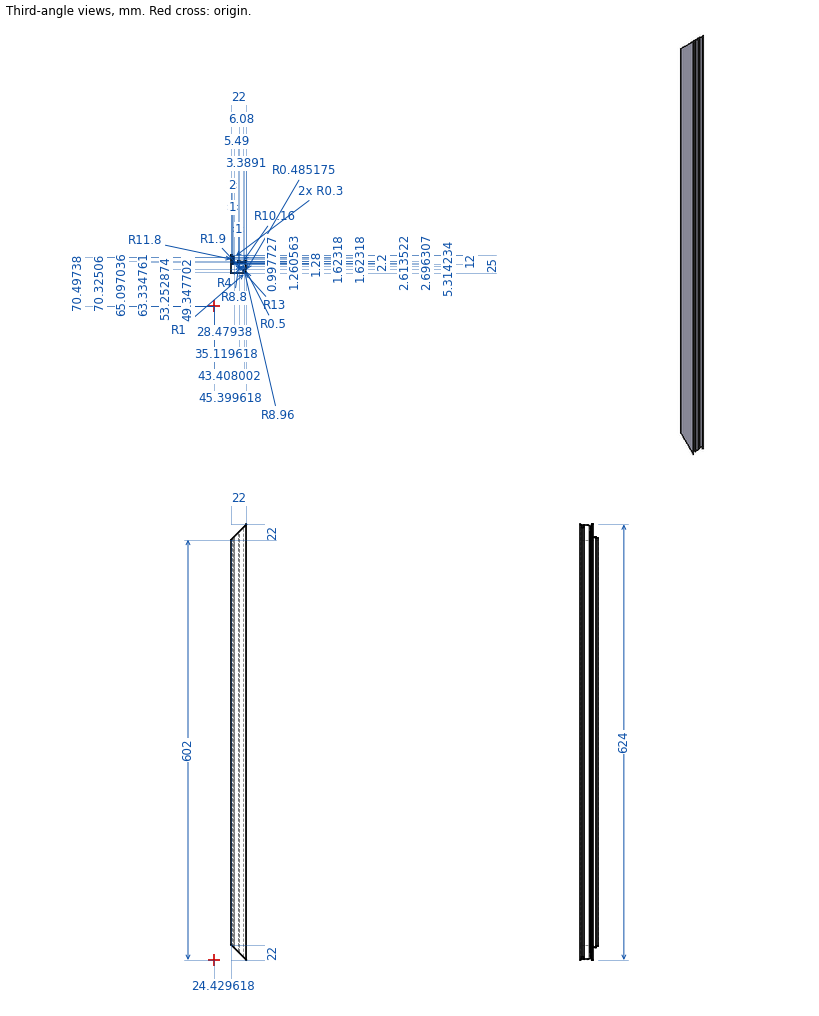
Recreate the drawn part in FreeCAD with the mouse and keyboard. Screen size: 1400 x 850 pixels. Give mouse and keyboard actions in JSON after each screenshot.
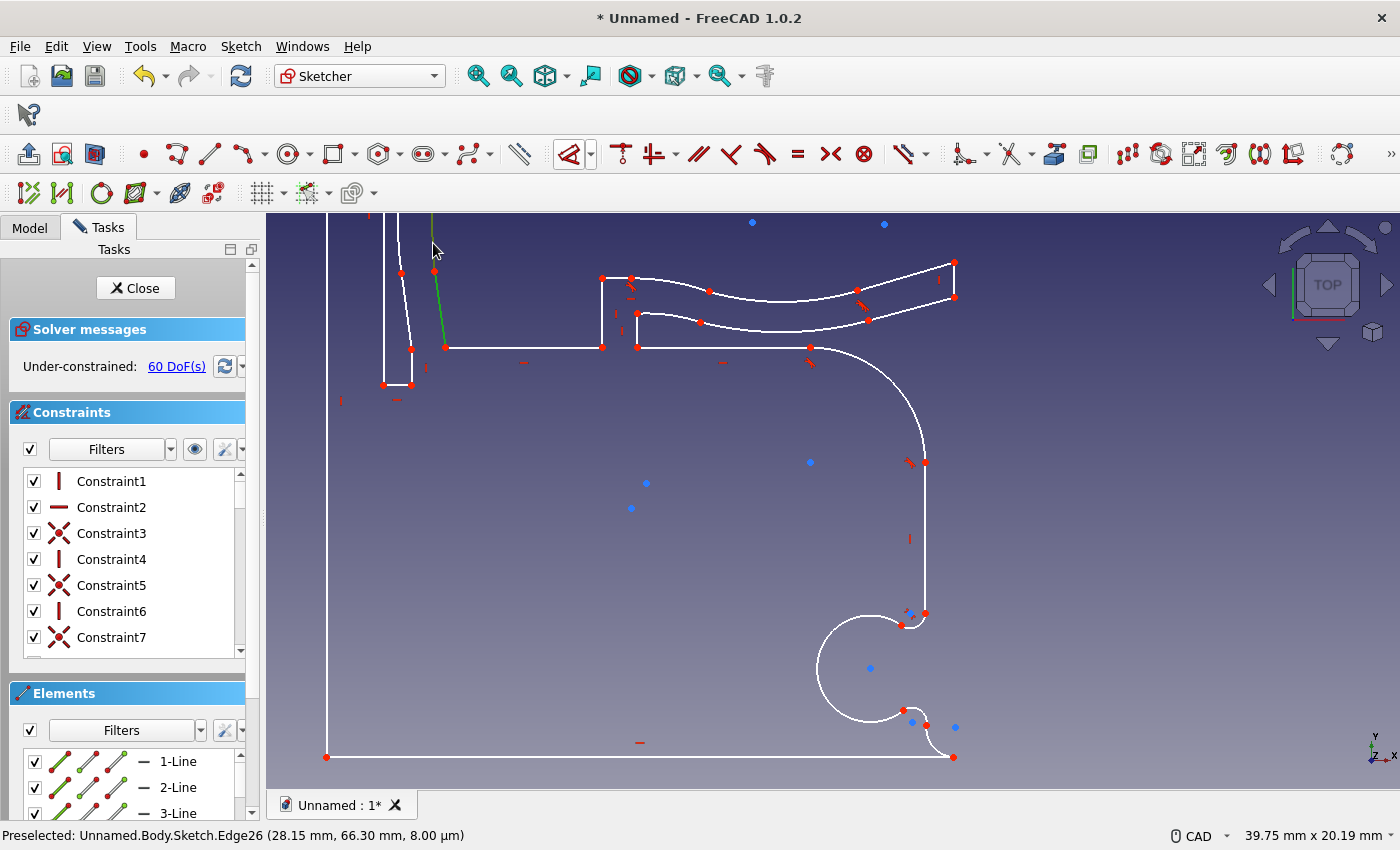
{"action": "left_click", "coordinate": [765, 154]}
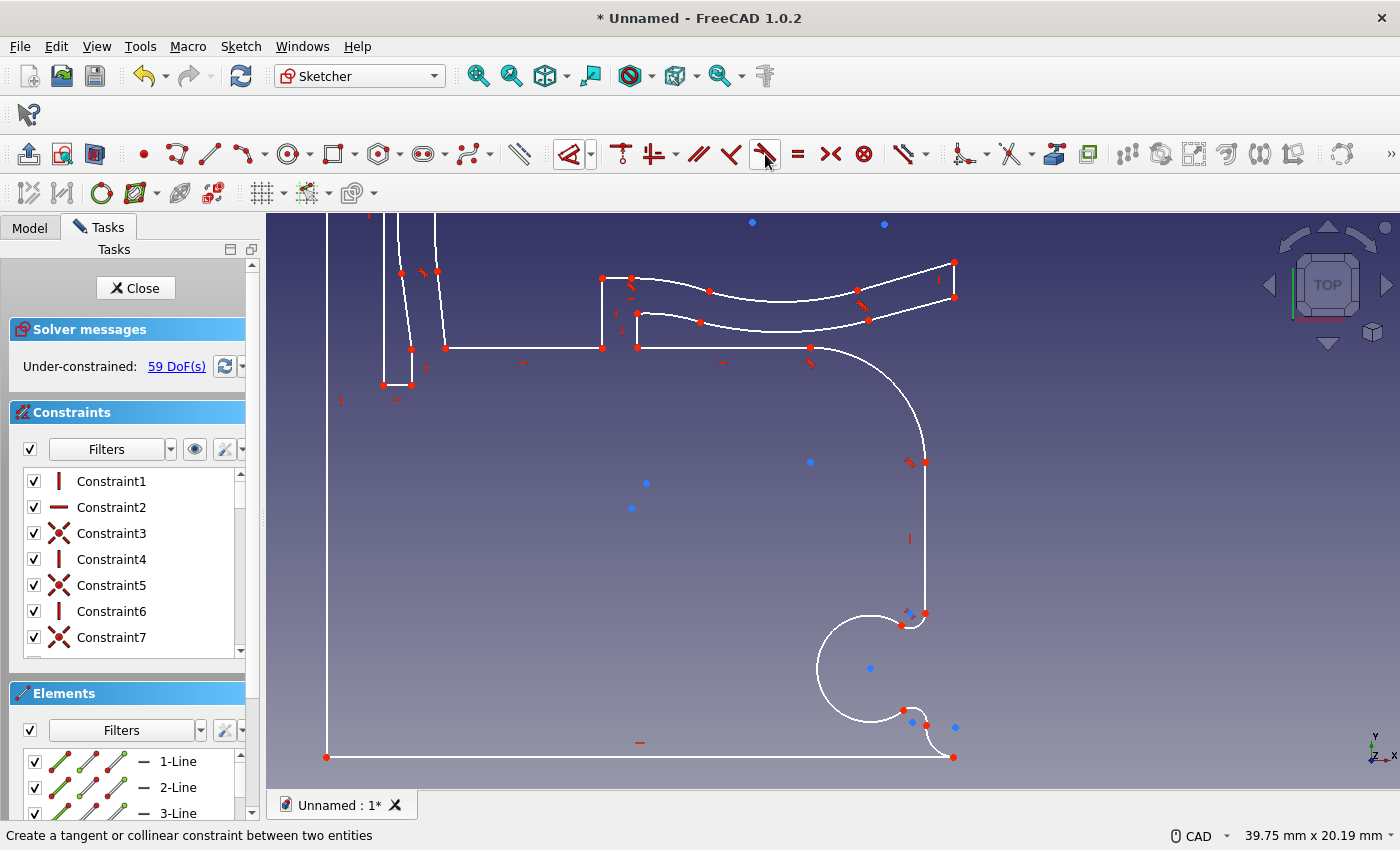
{"action": "scroll", "coordinate": [916, 625], "scroll_direction": "down", "scroll_amount": 3}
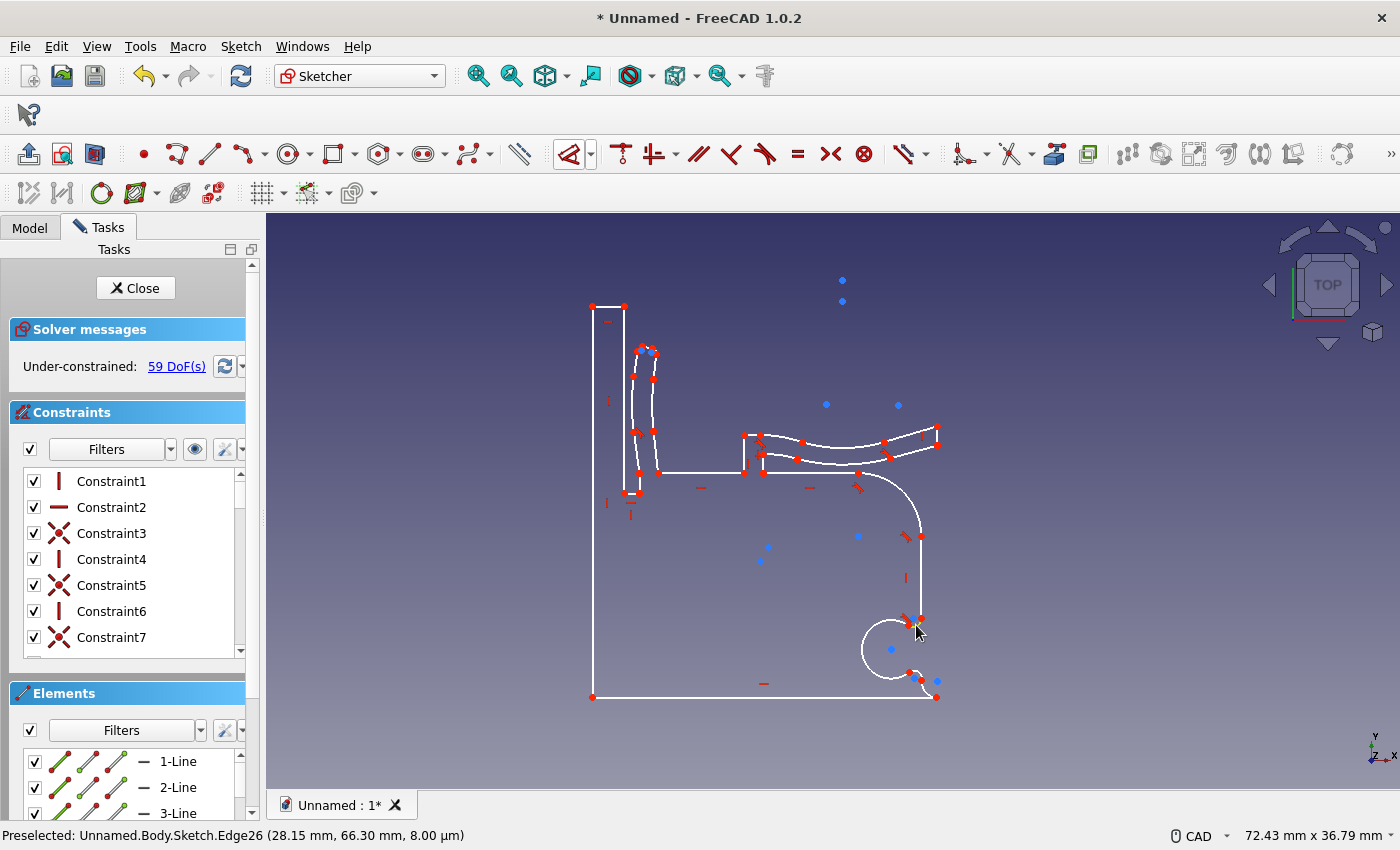
{"action": "scroll", "coordinate": [654, 372], "scroll_direction": "up", "scroll_amount": 4}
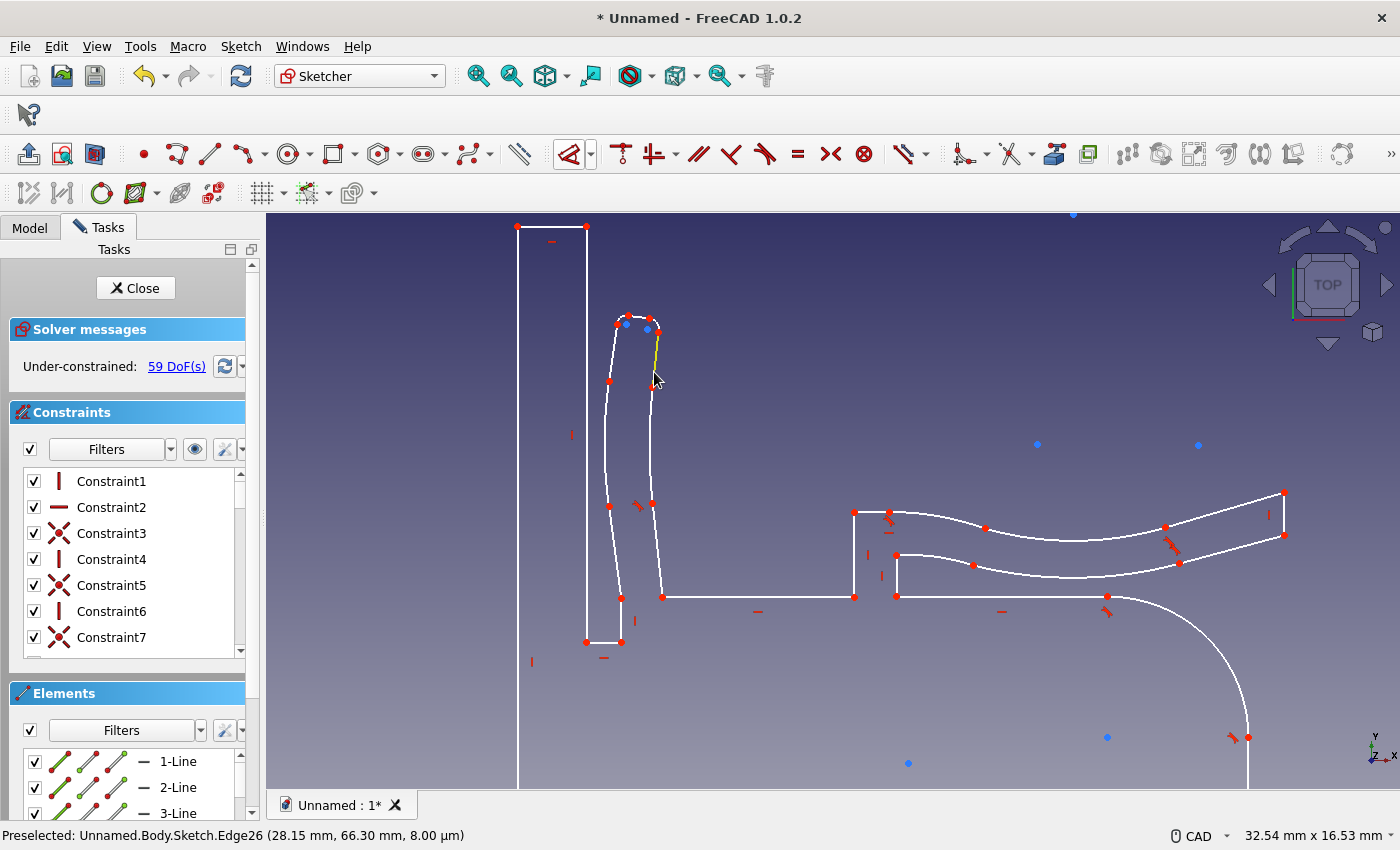
{"action": "left_click", "coordinate": [654, 371]}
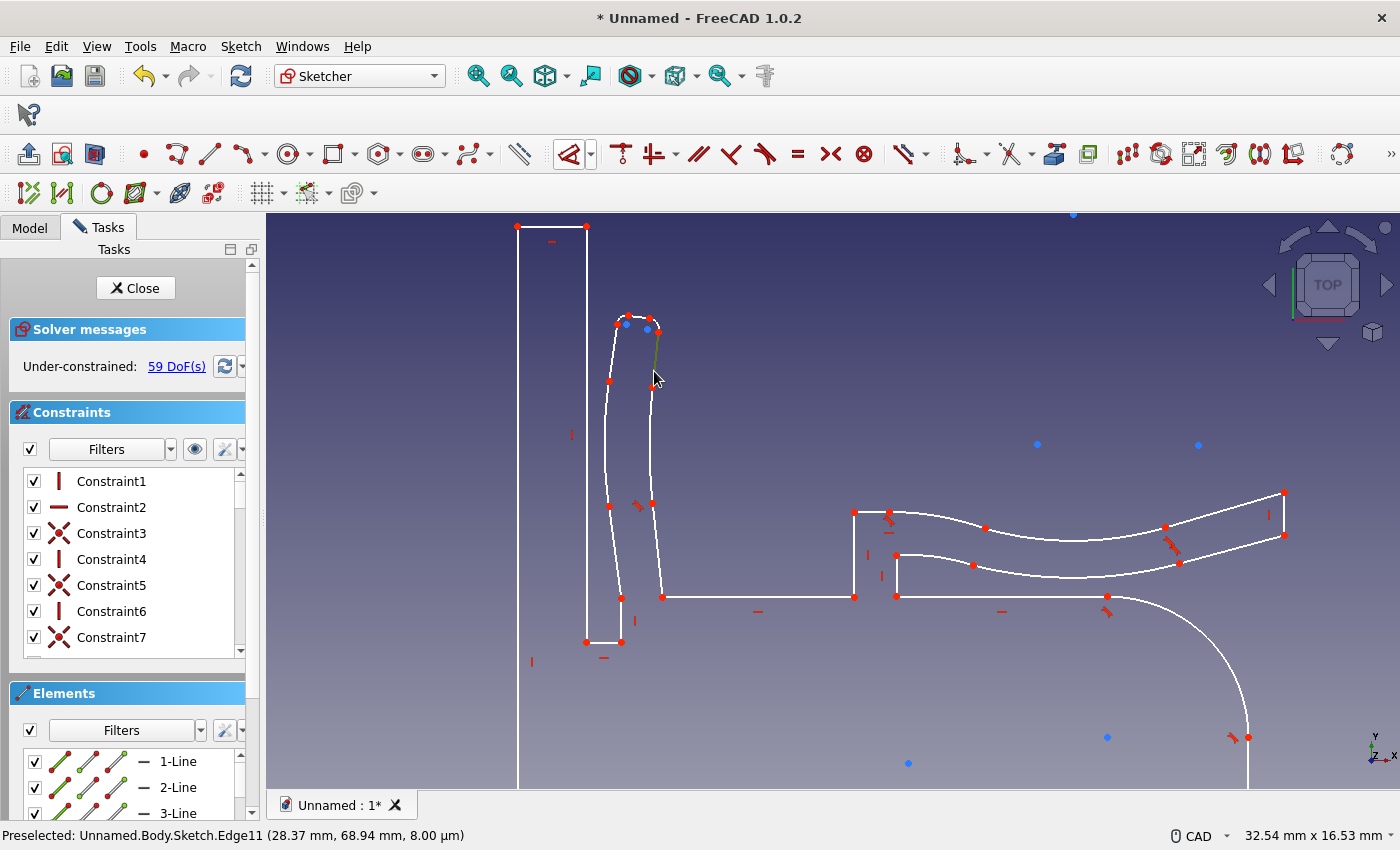
{"action": "left_click", "coordinate": [650, 423]}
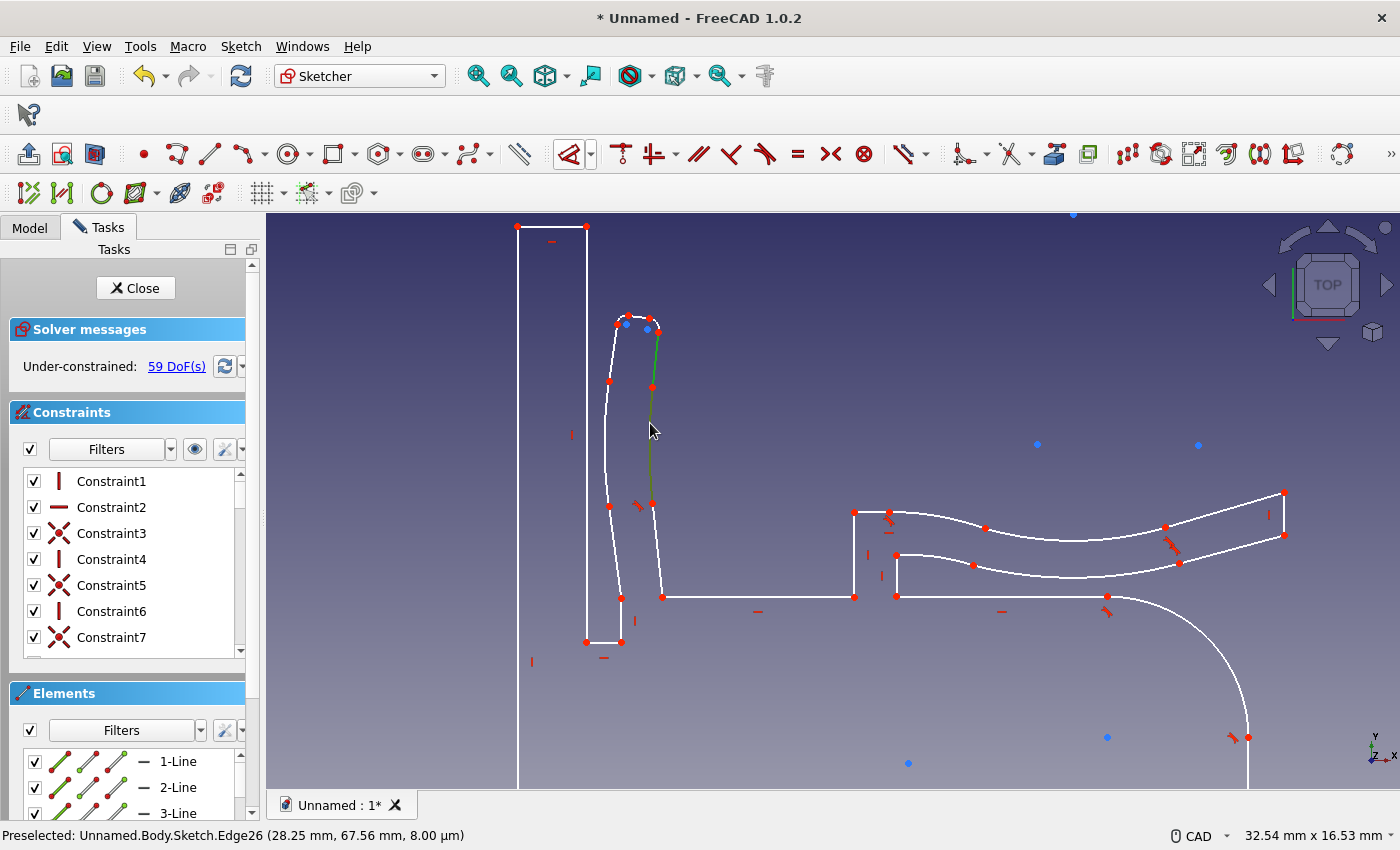
{"action": "key", "text": "t"}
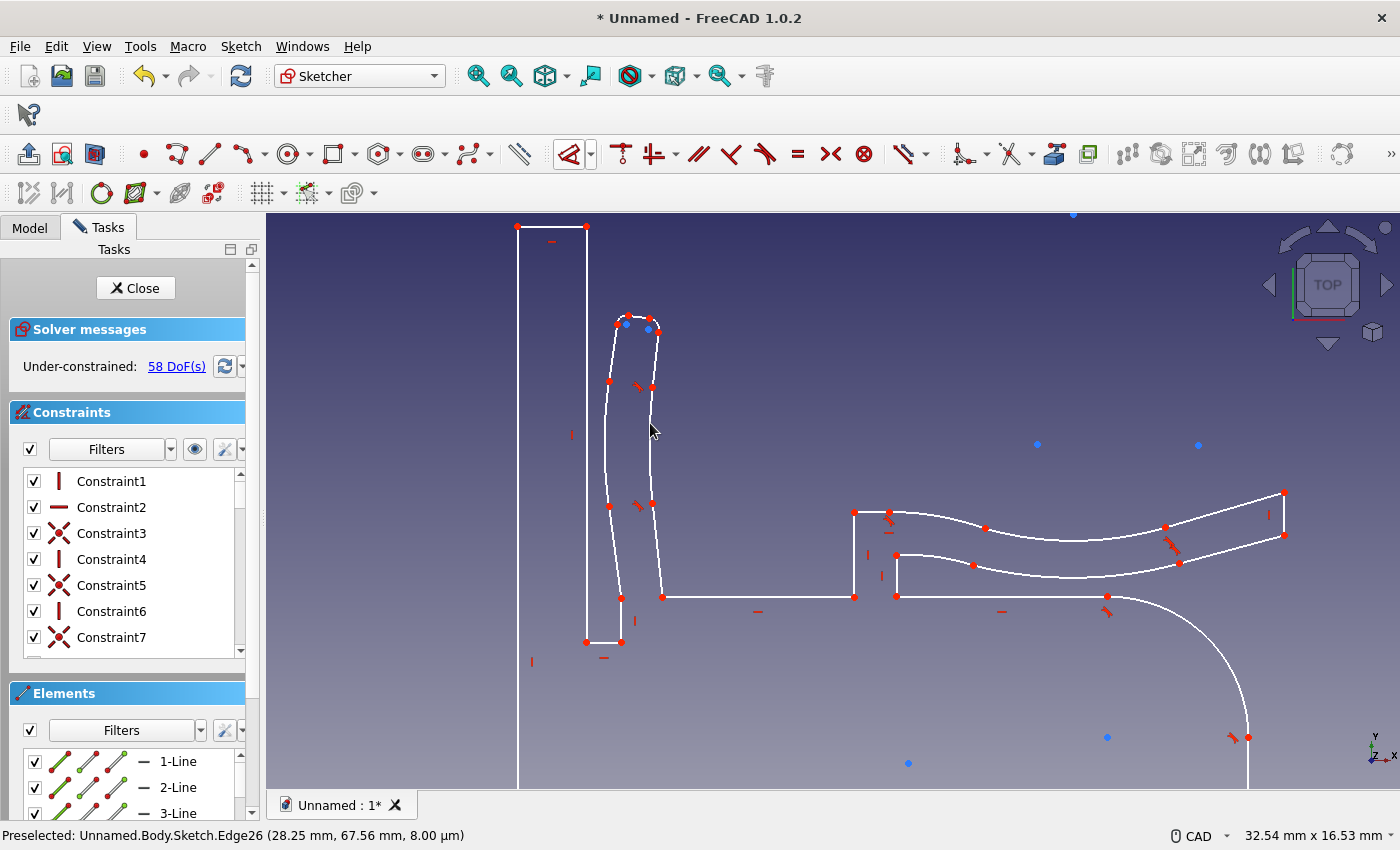
{"action": "left_click", "coordinate": [654, 371]}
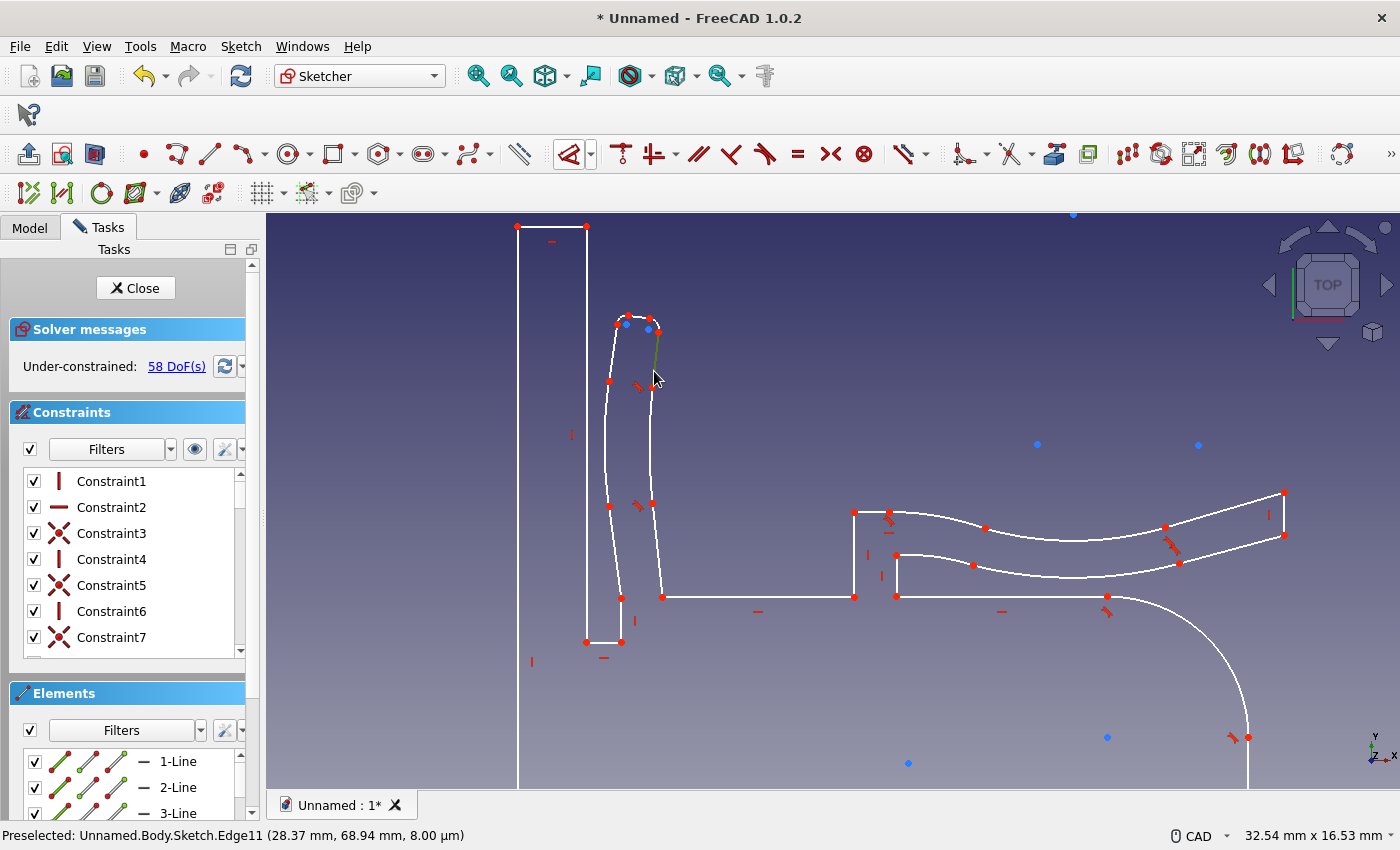
{"action": "scroll", "coordinate": [657, 323], "scroll_direction": "up", "scroll_amount": 3}